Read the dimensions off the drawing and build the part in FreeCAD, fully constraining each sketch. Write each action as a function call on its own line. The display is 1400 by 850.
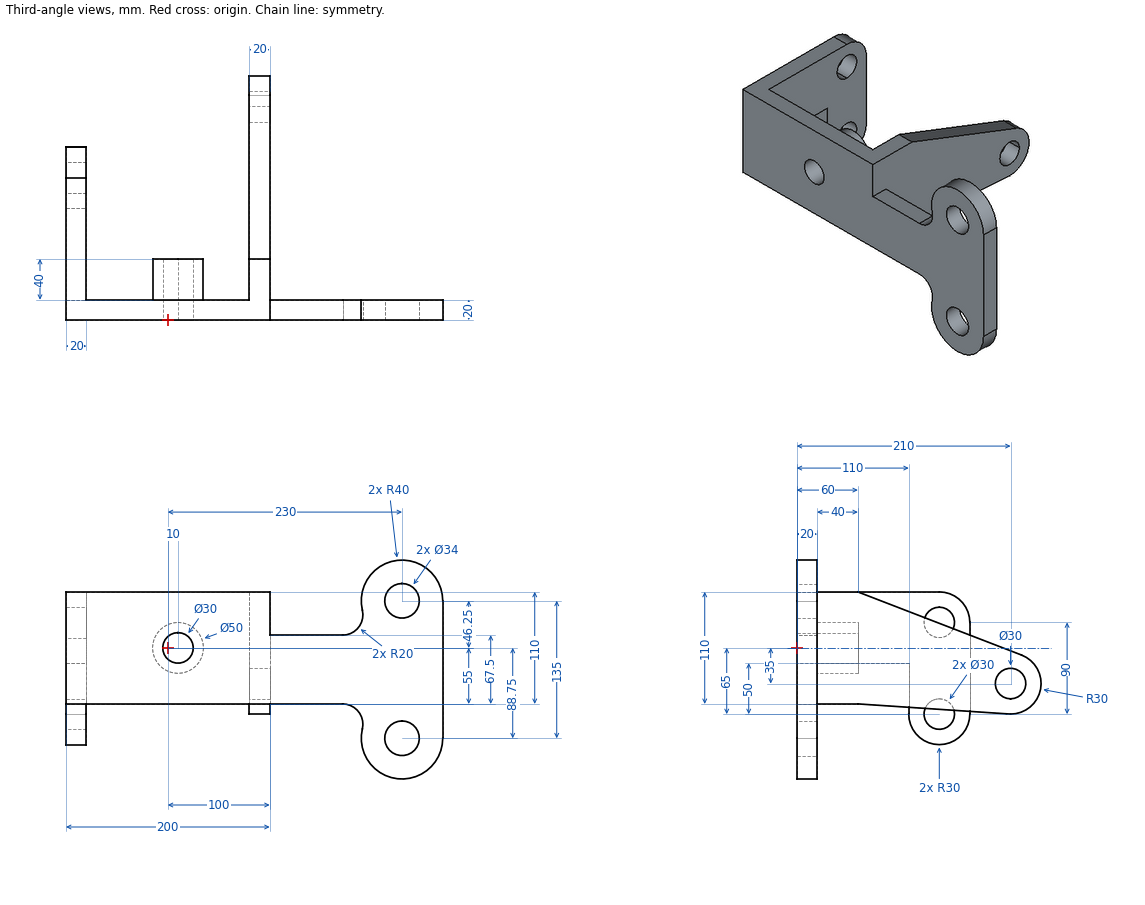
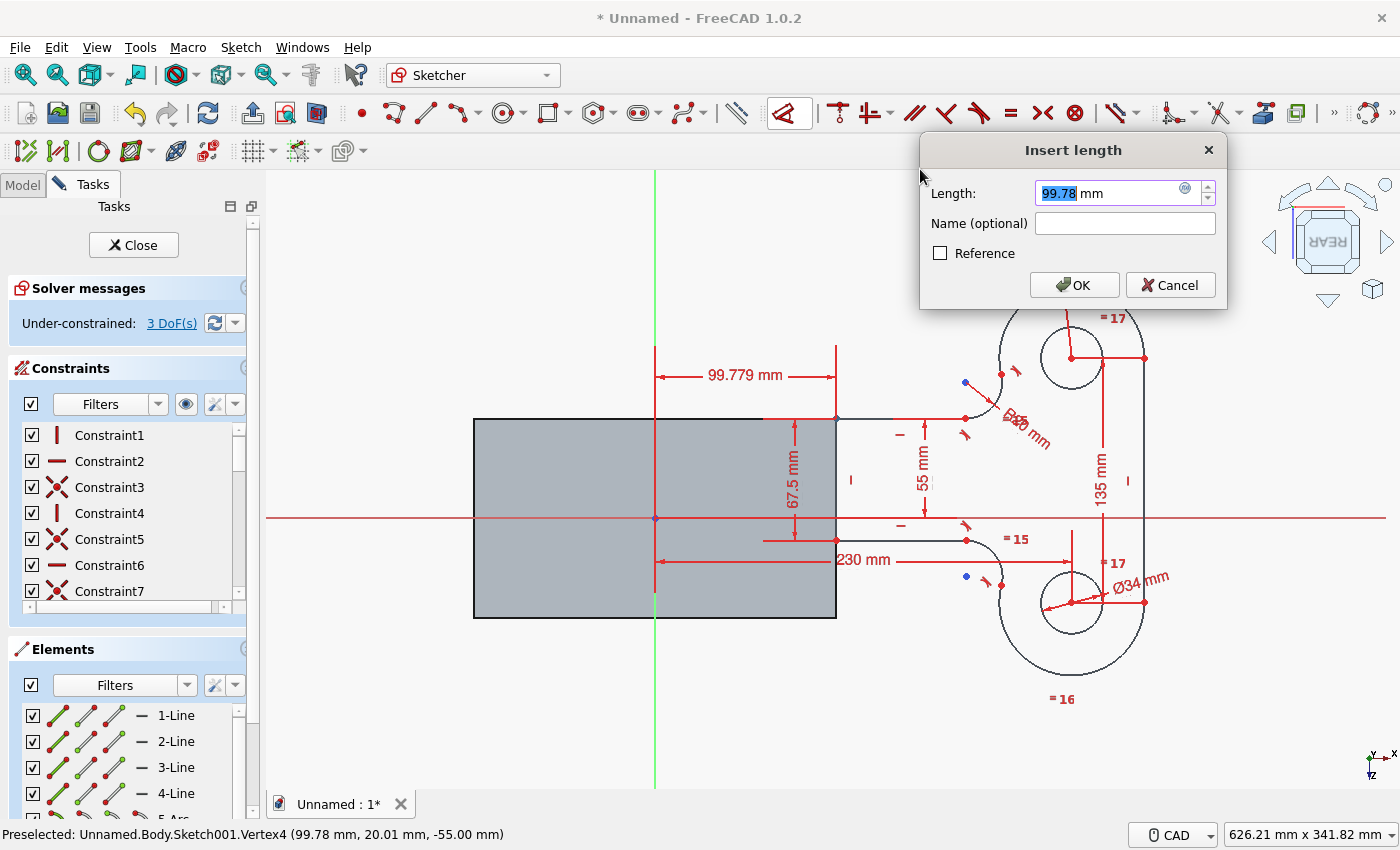
text(100)
key(Return)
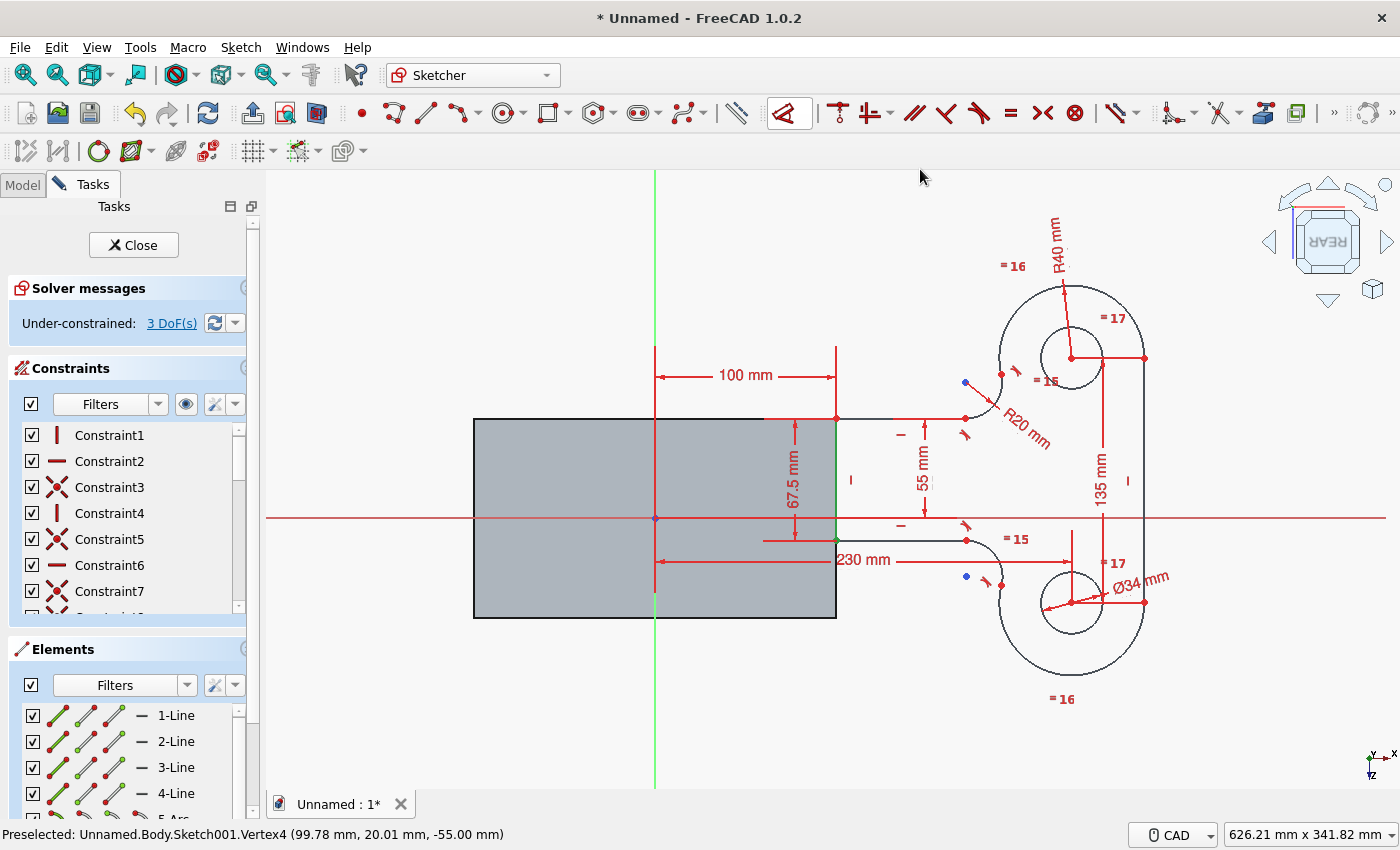
click(1072, 603)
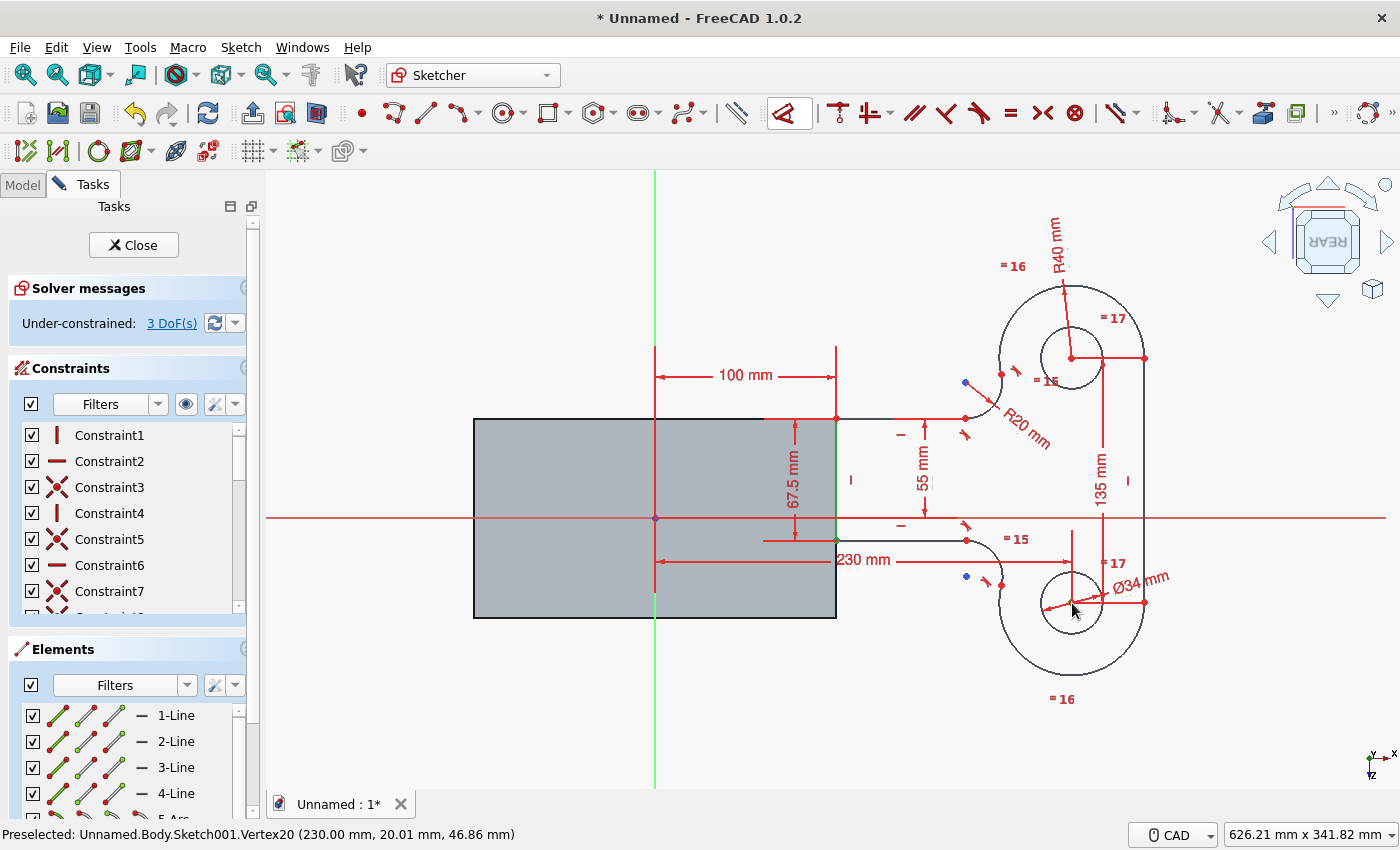
key(i)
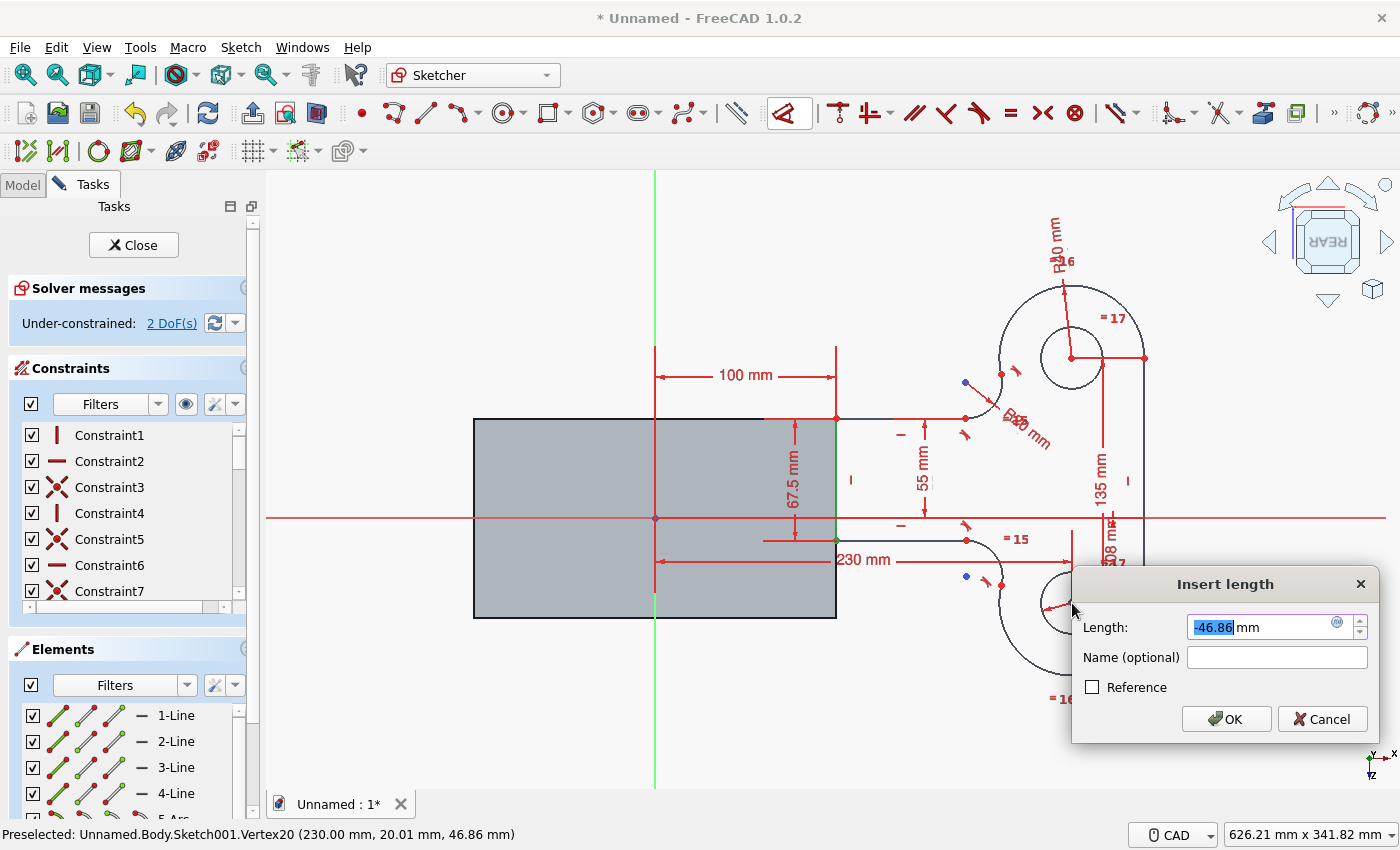
text(-46.25)
key(Return)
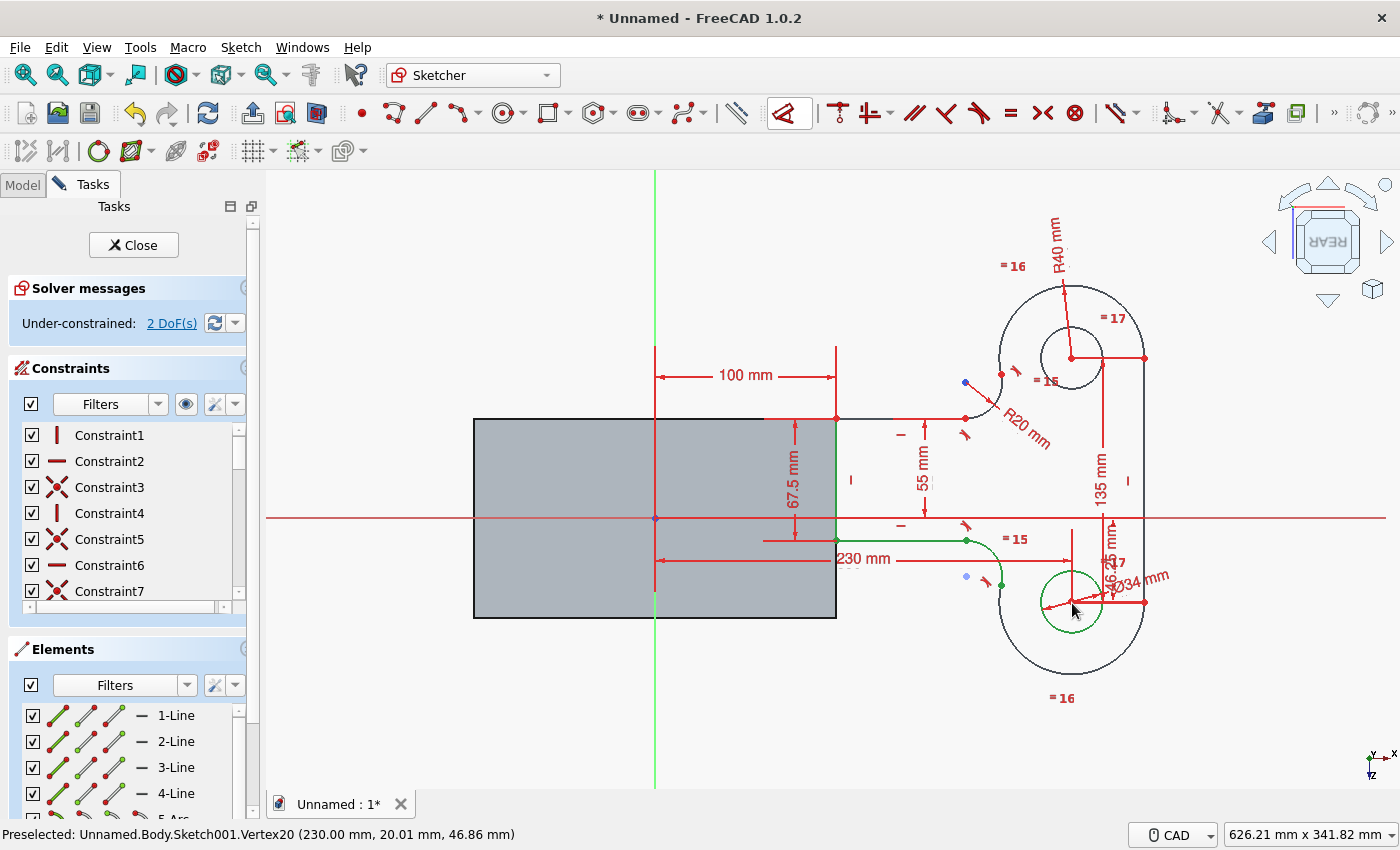
click(1072, 358)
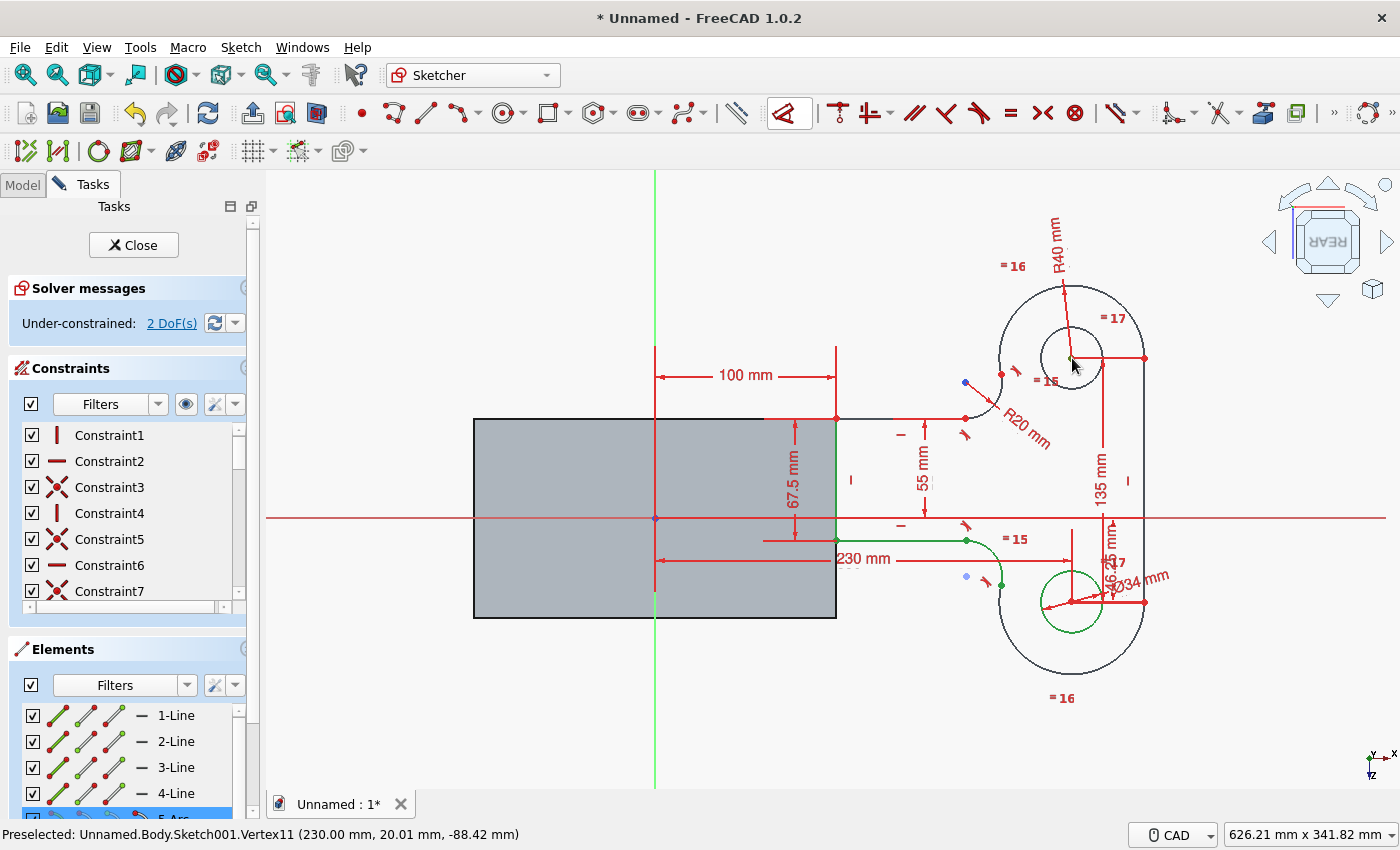
key(i)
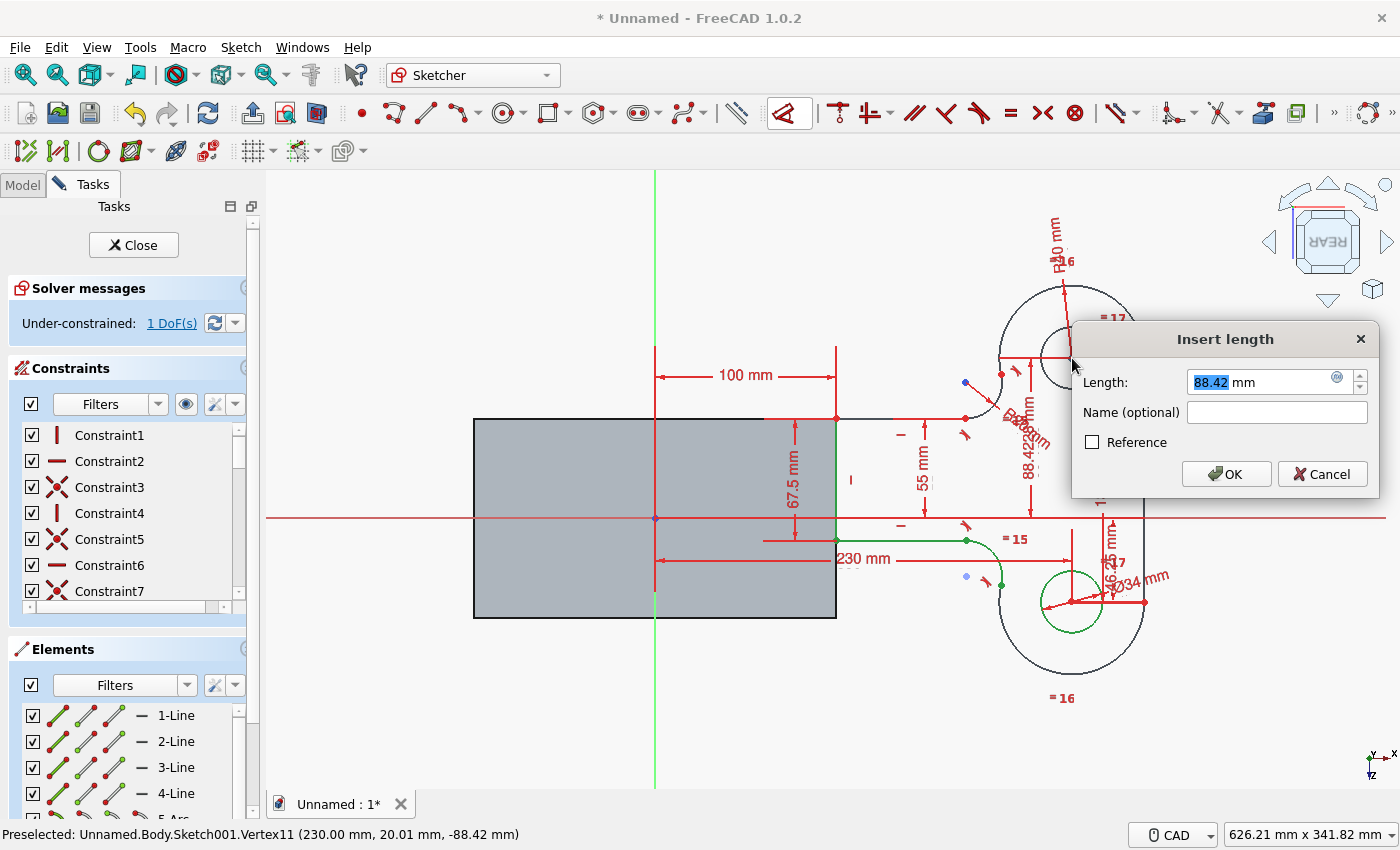
text(88.75)
key(Return)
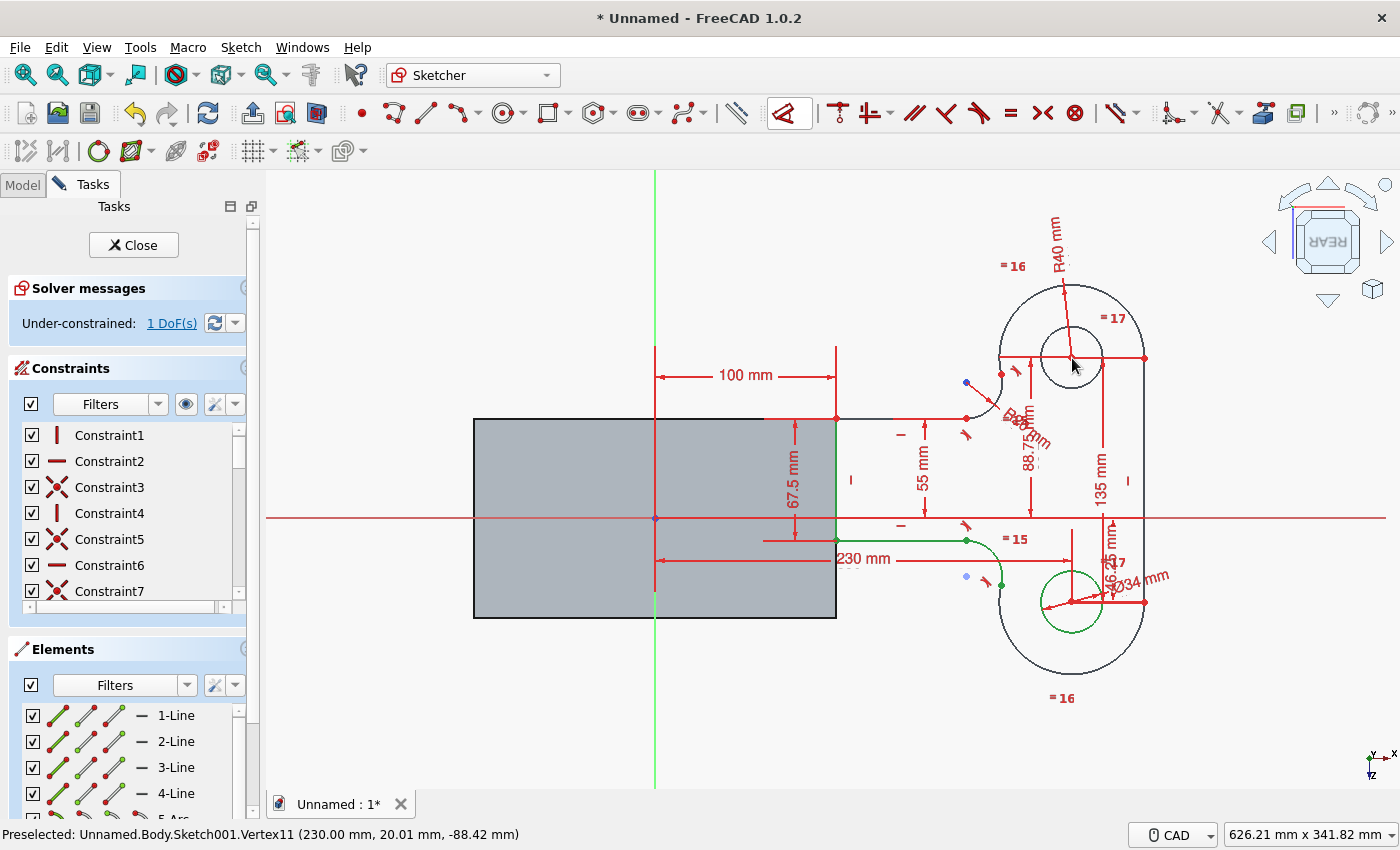
click(1144, 603)